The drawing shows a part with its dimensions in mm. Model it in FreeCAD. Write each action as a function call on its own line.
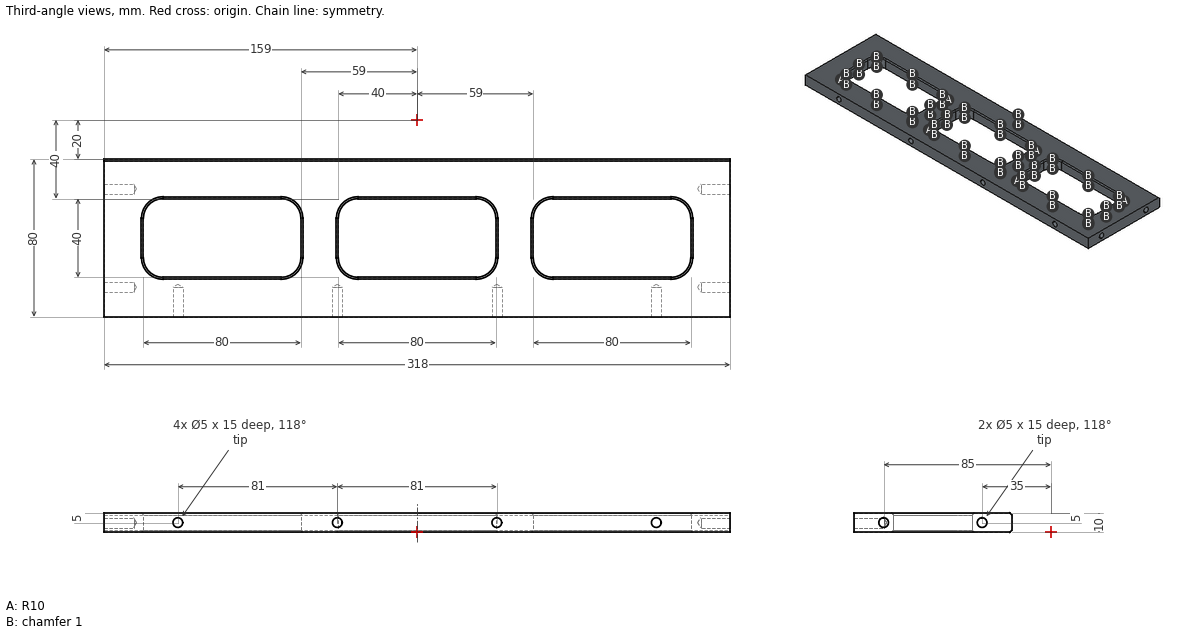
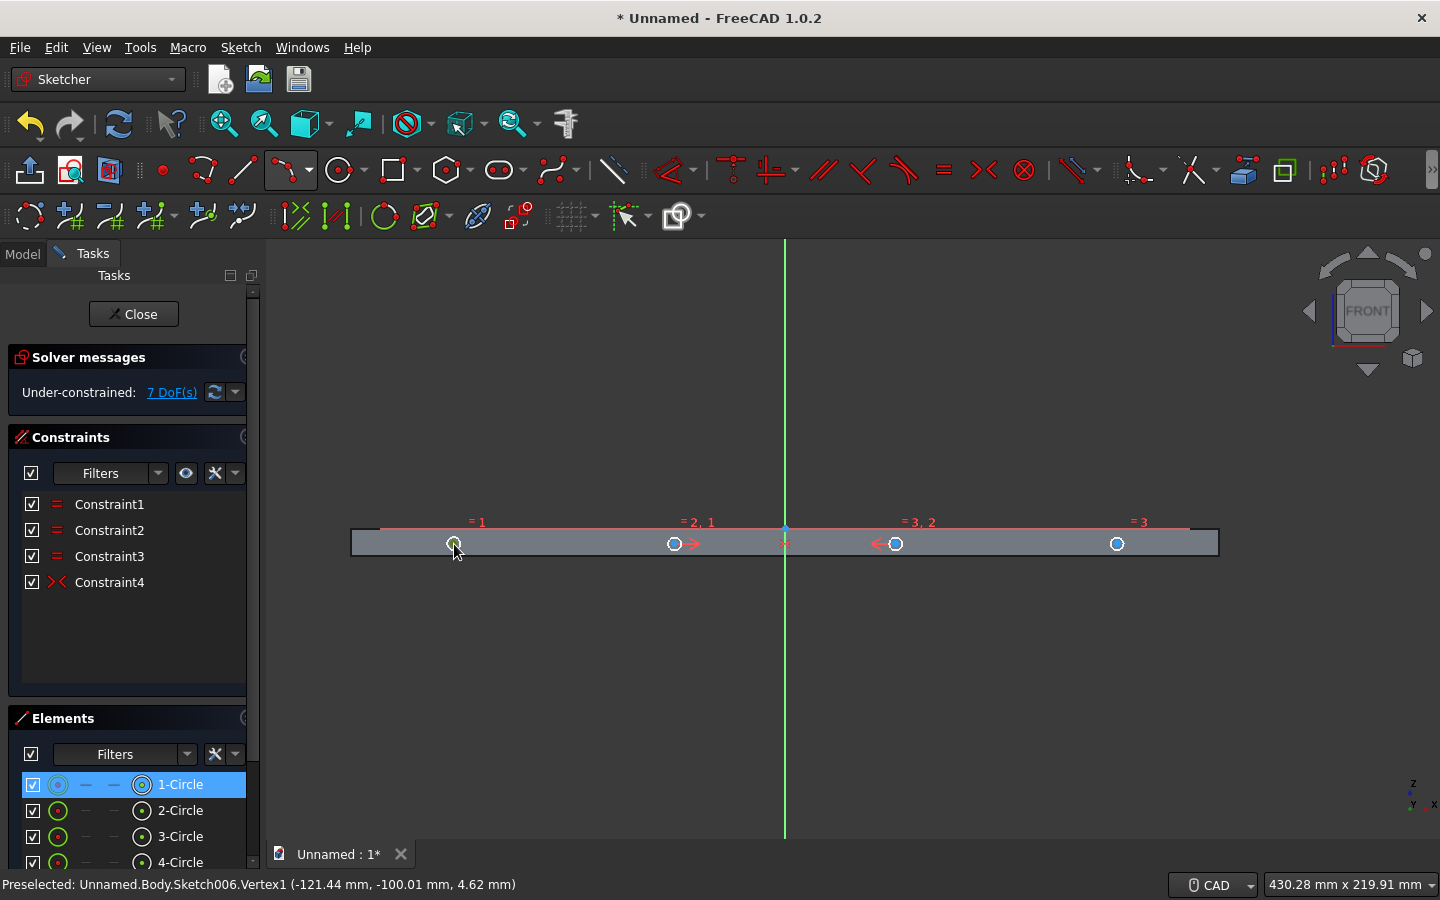
click(1117, 544)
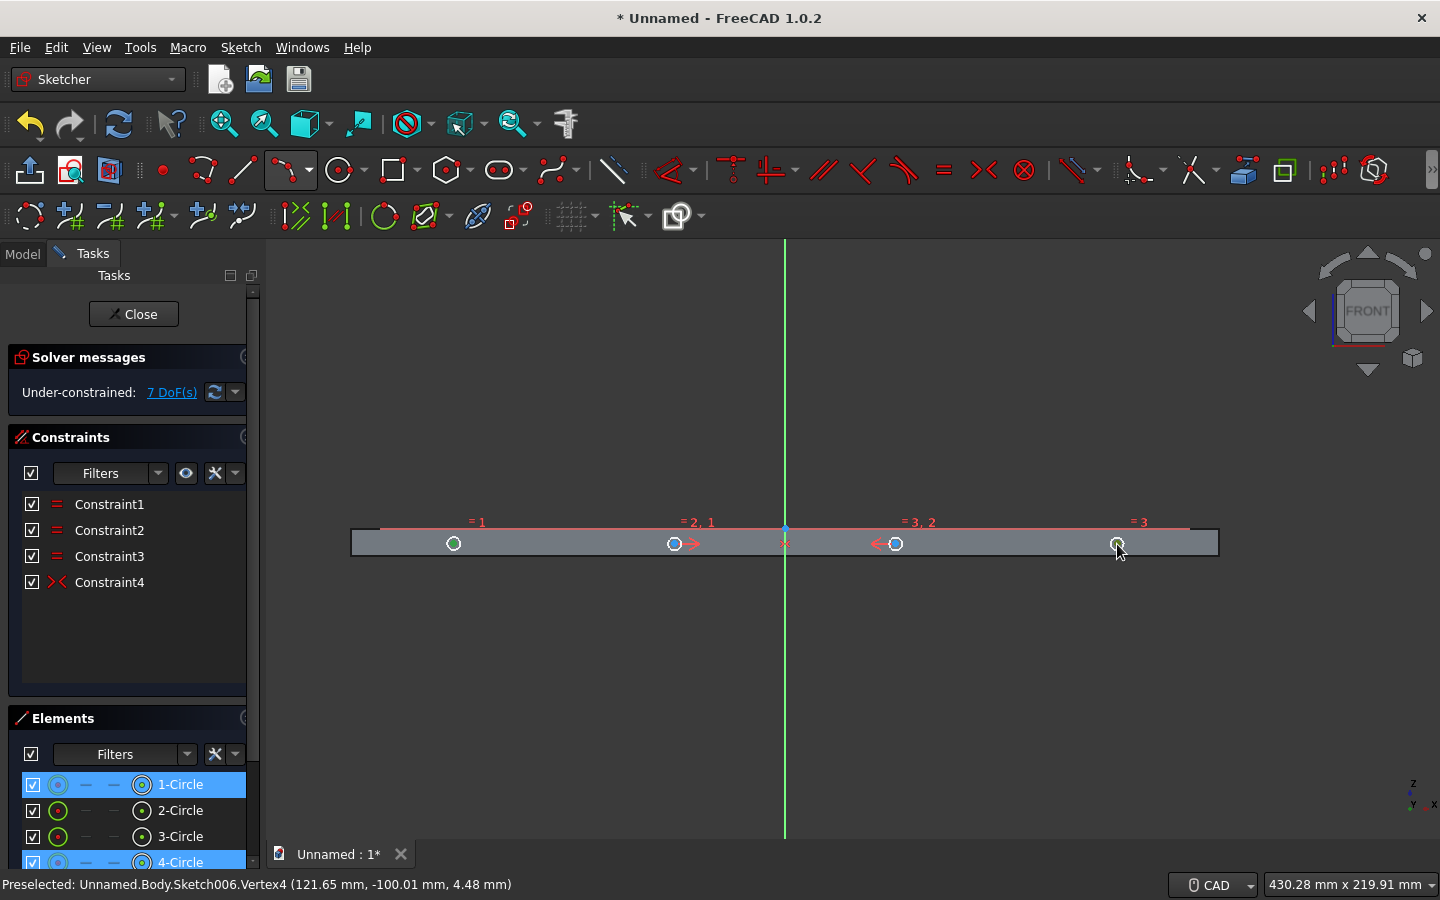
click(785, 772)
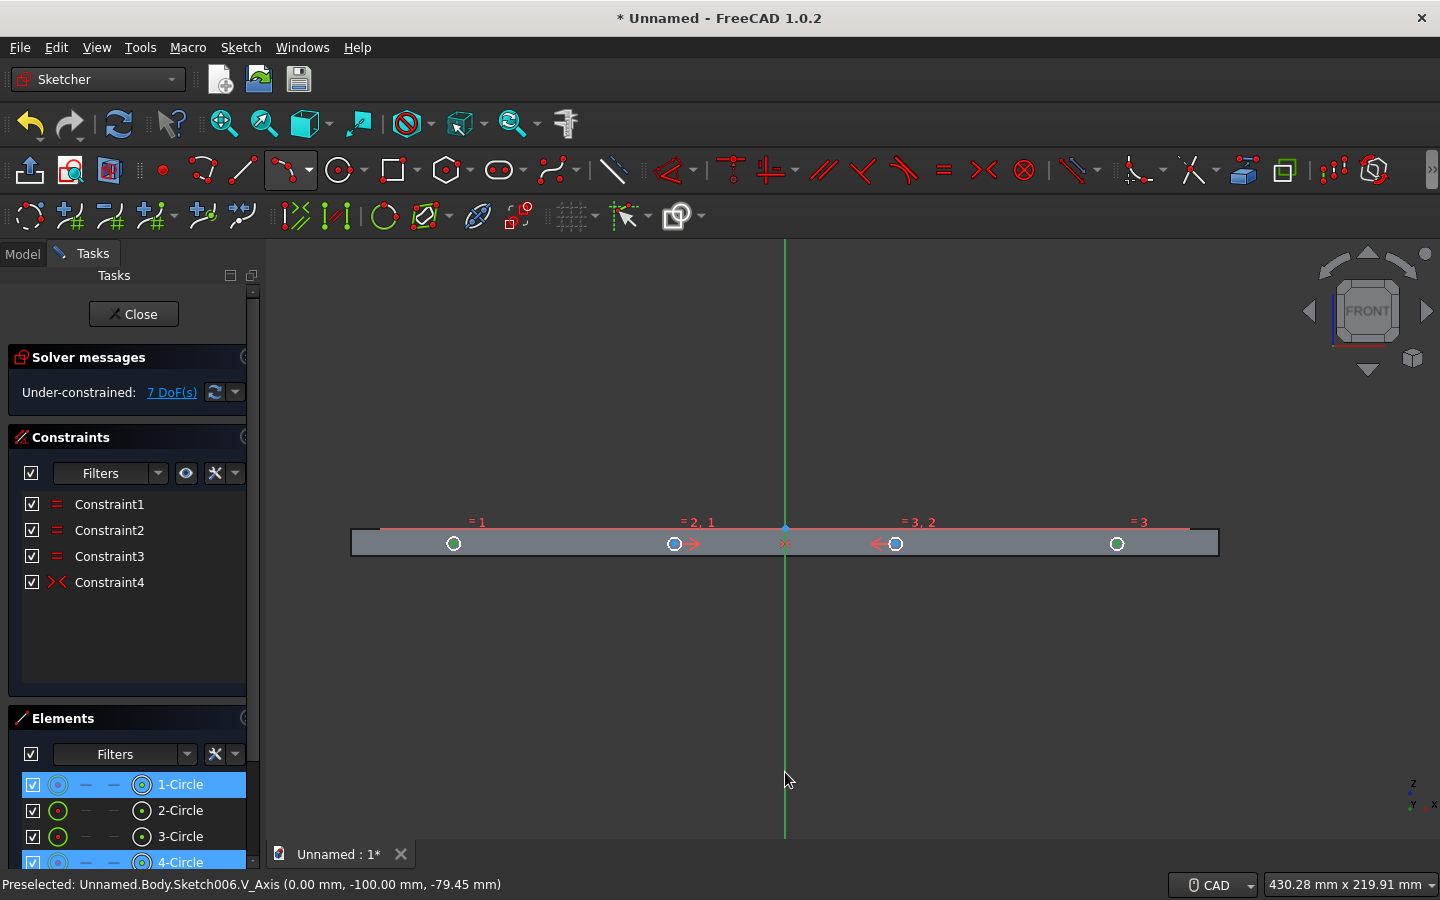
key(s)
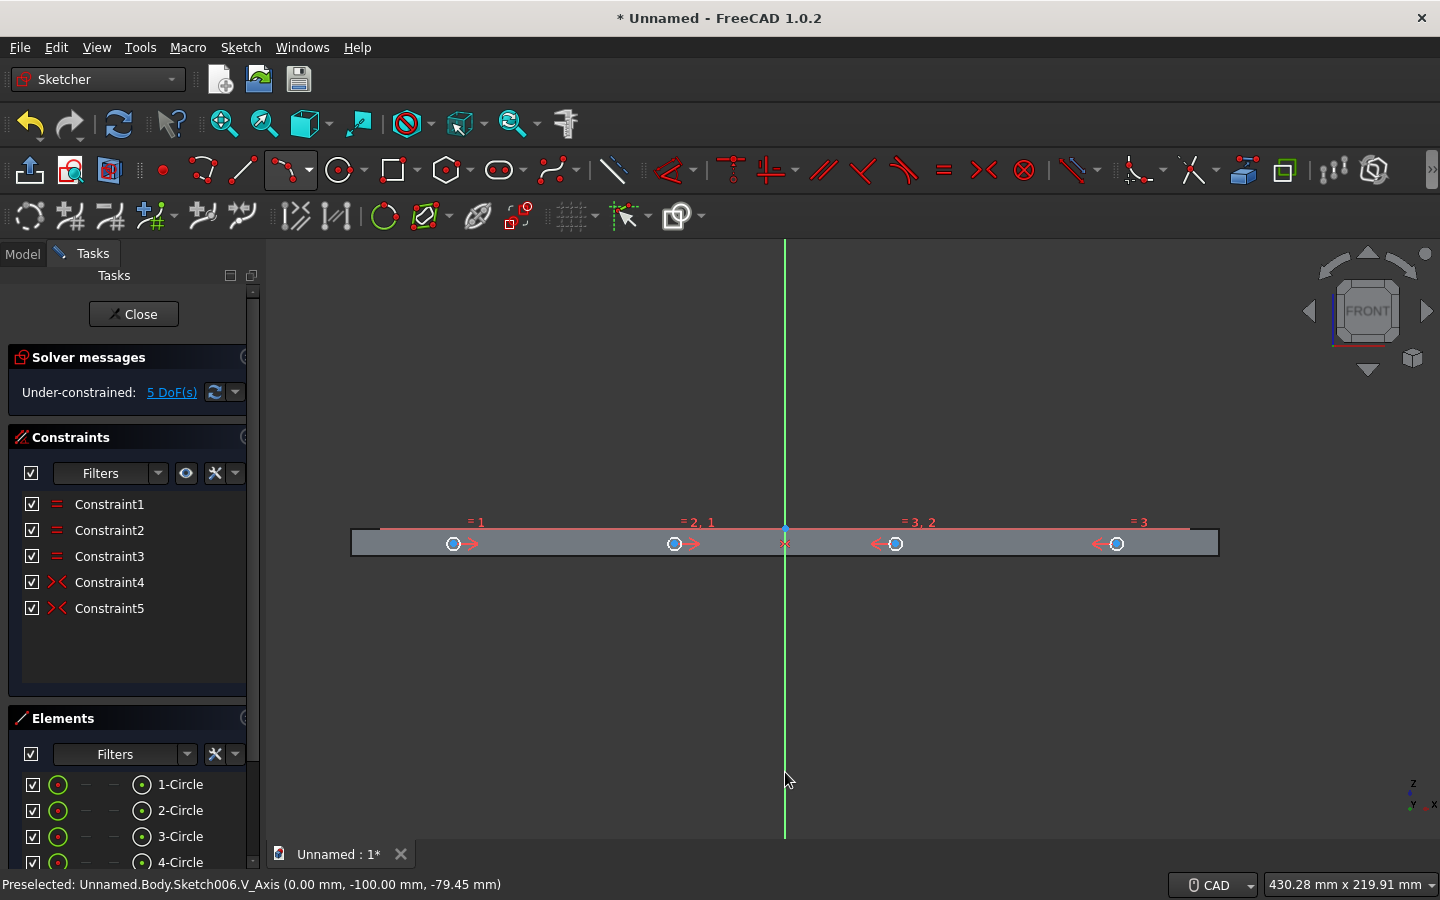
click(668, 170)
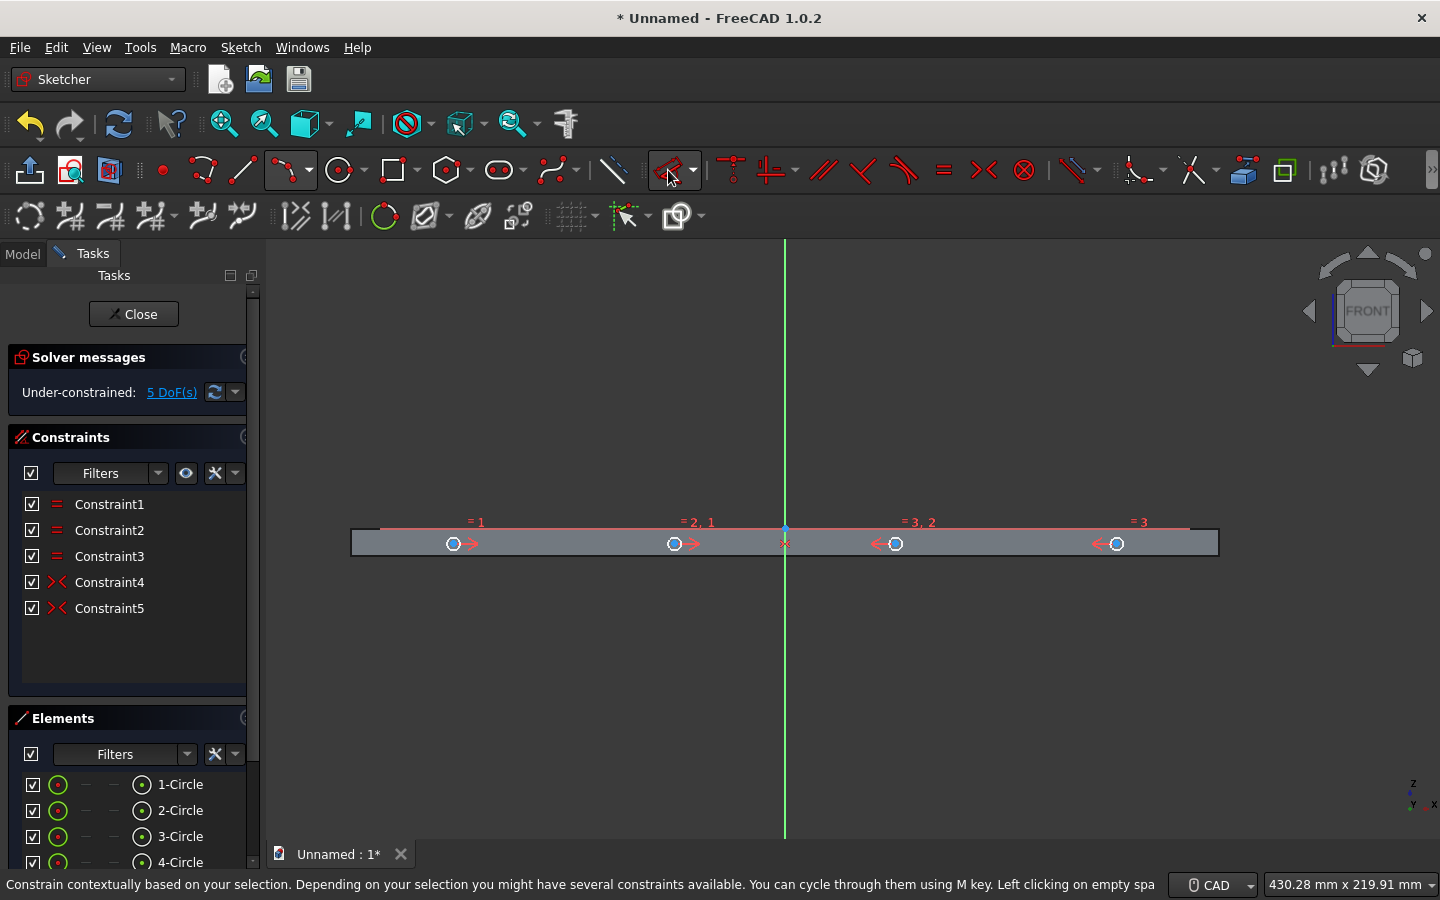
scroll(447, 544, up, 6)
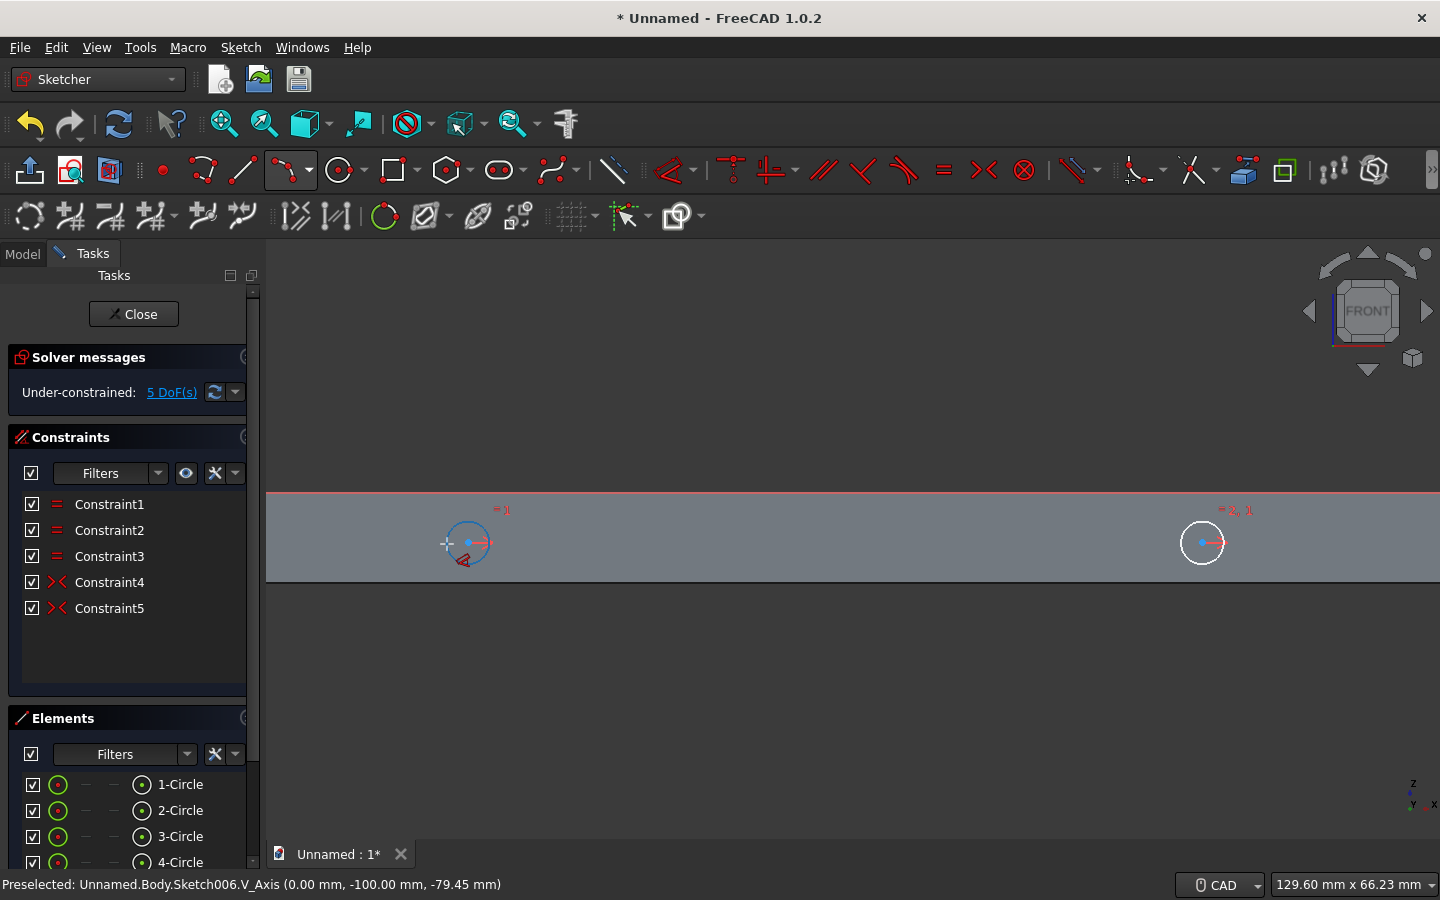
click(447, 542)
click(415, 541)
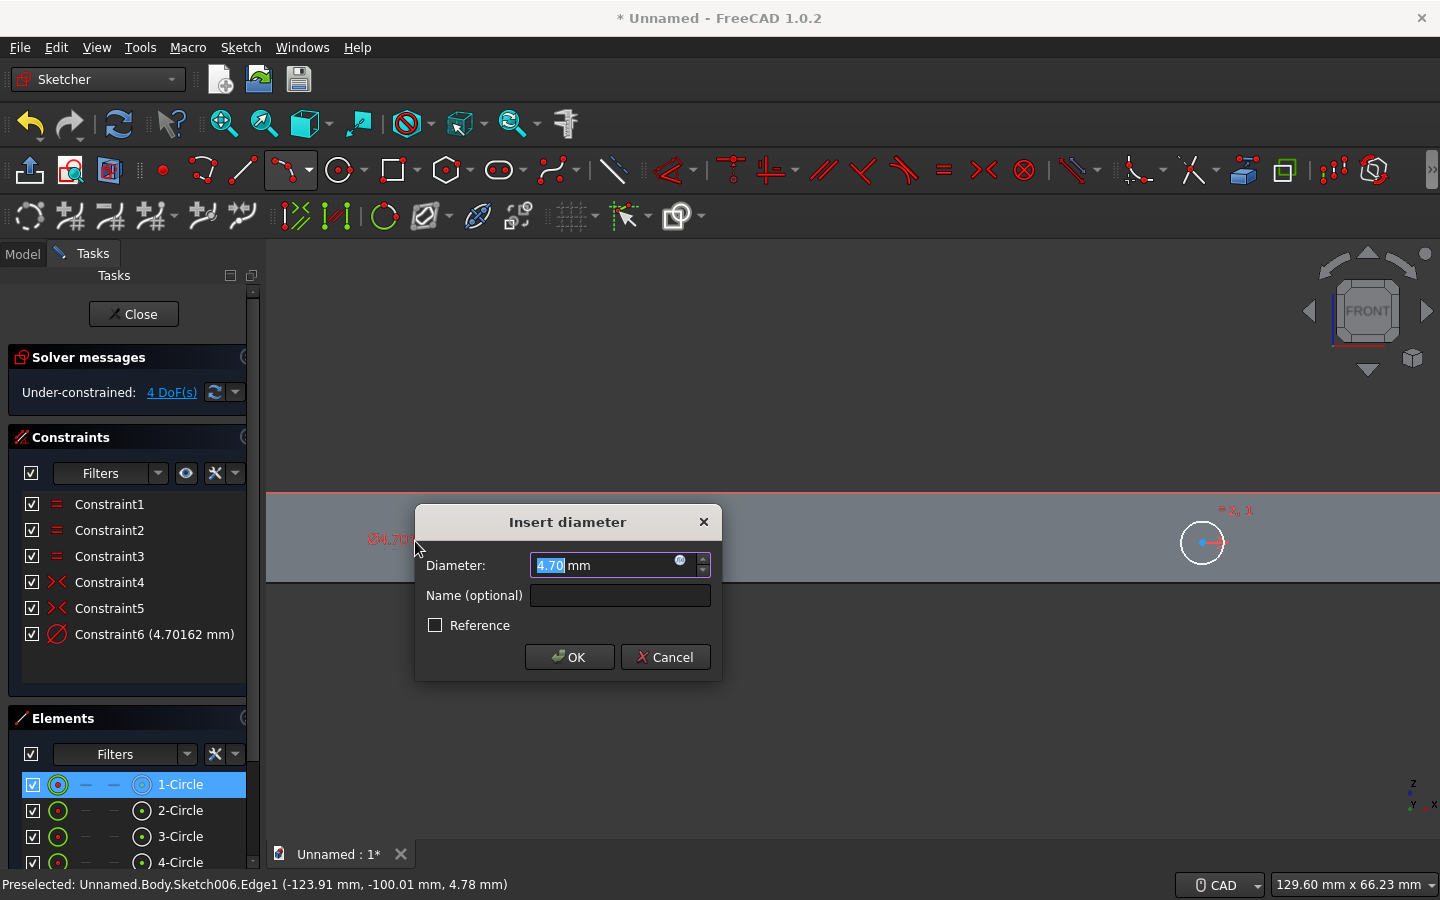
text(5)
key(Return)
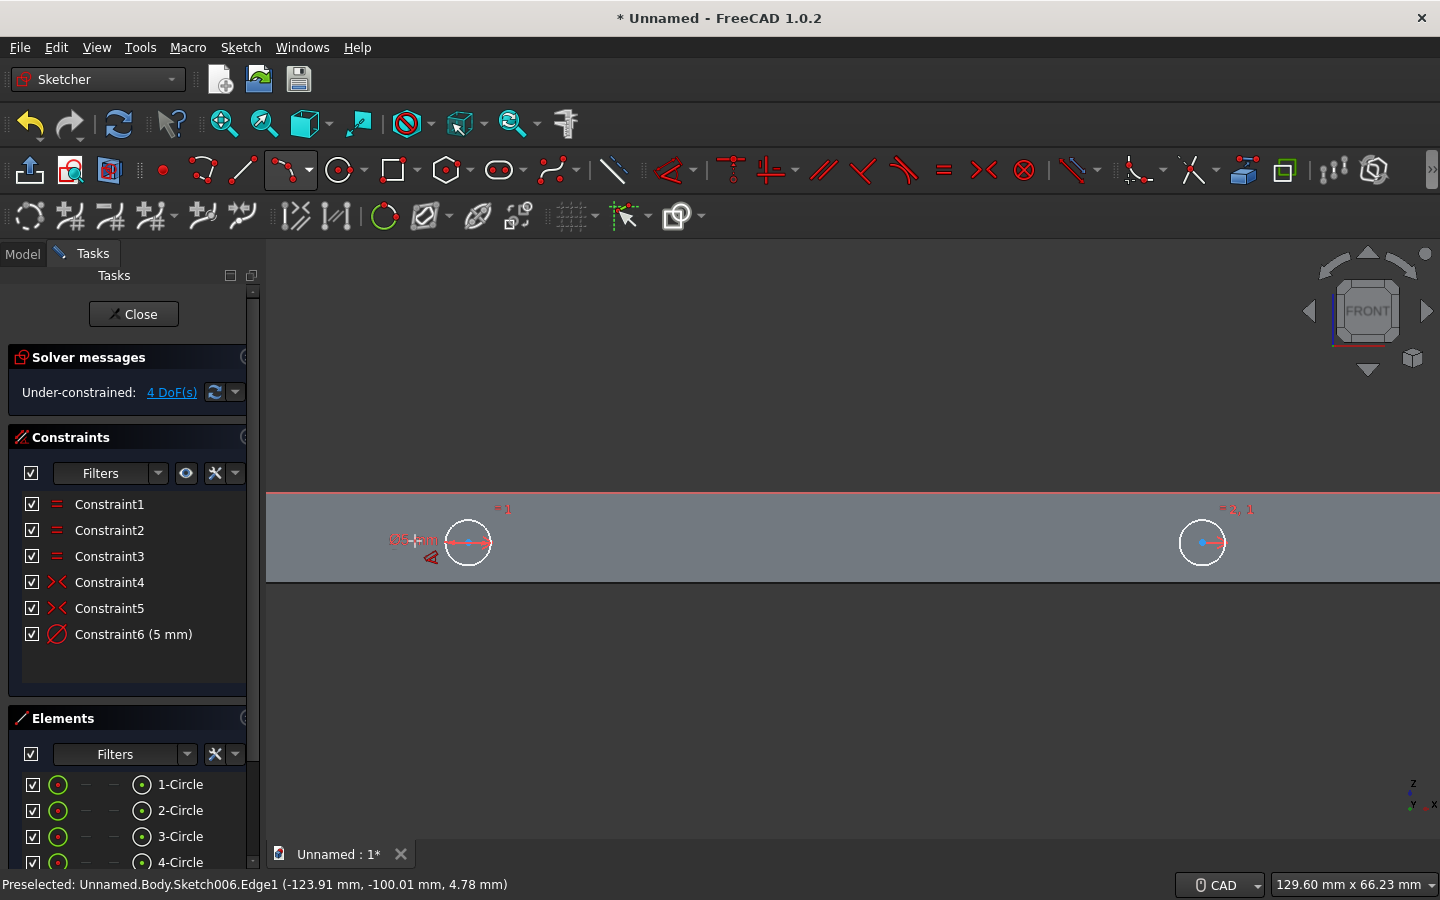
click(468, 543)
click(434, 518)